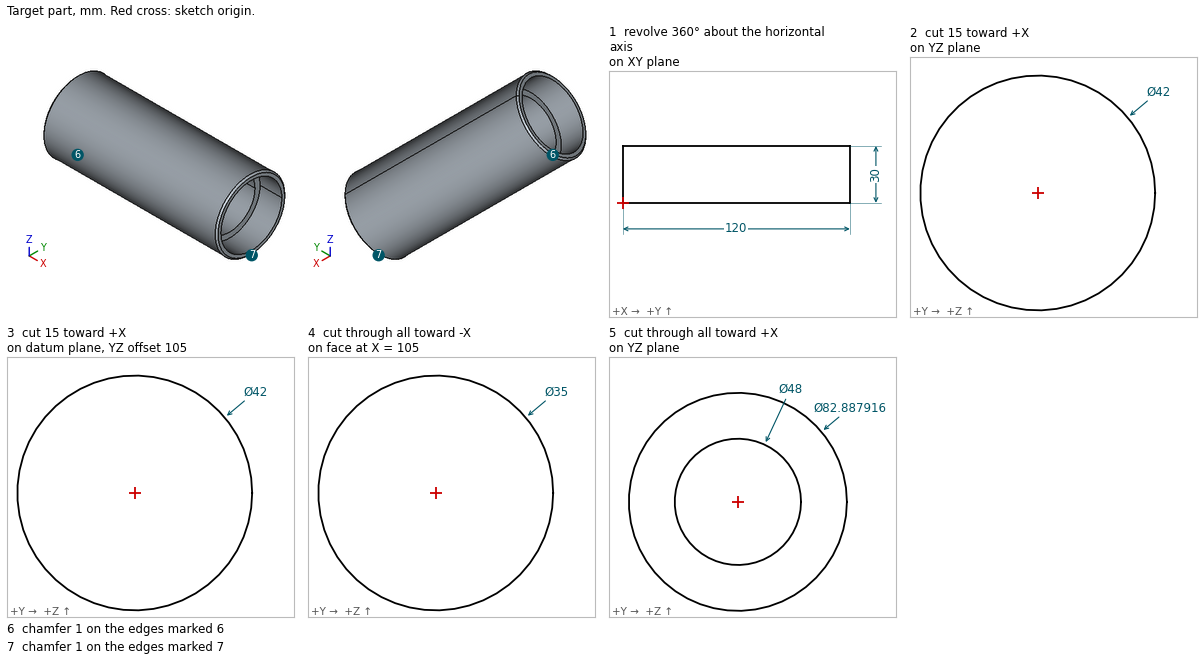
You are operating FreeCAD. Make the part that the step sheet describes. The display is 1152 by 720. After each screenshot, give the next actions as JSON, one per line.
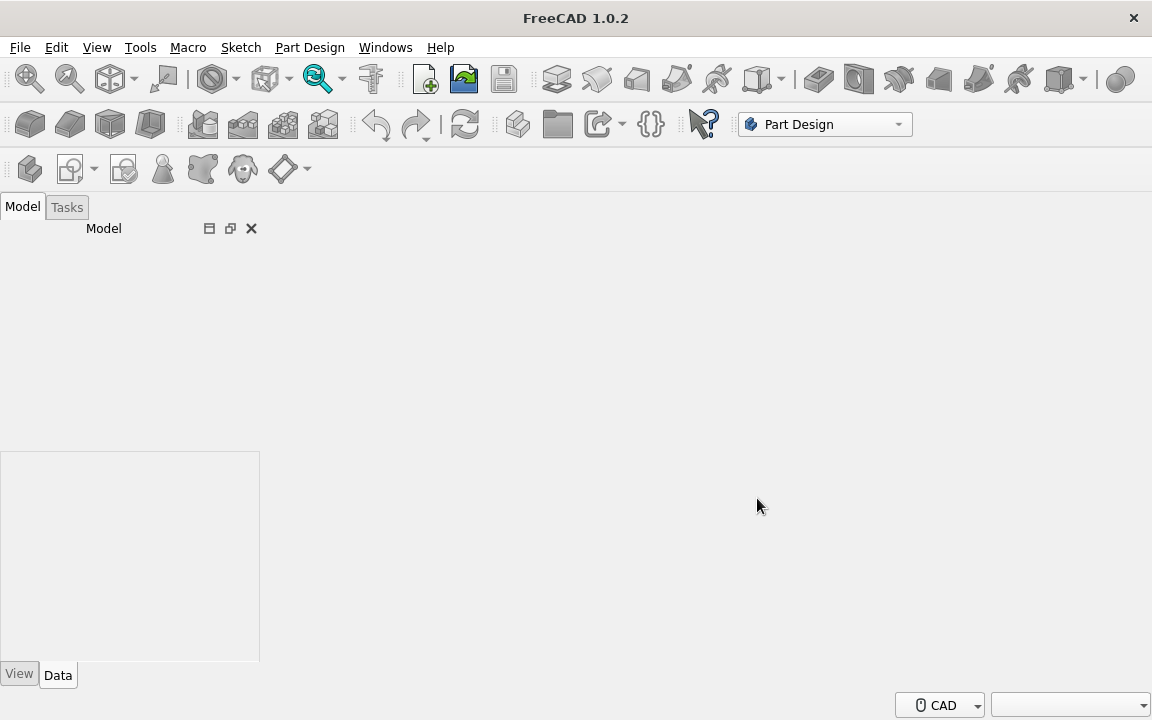
{"action": "key", "text": "ctrl+n"}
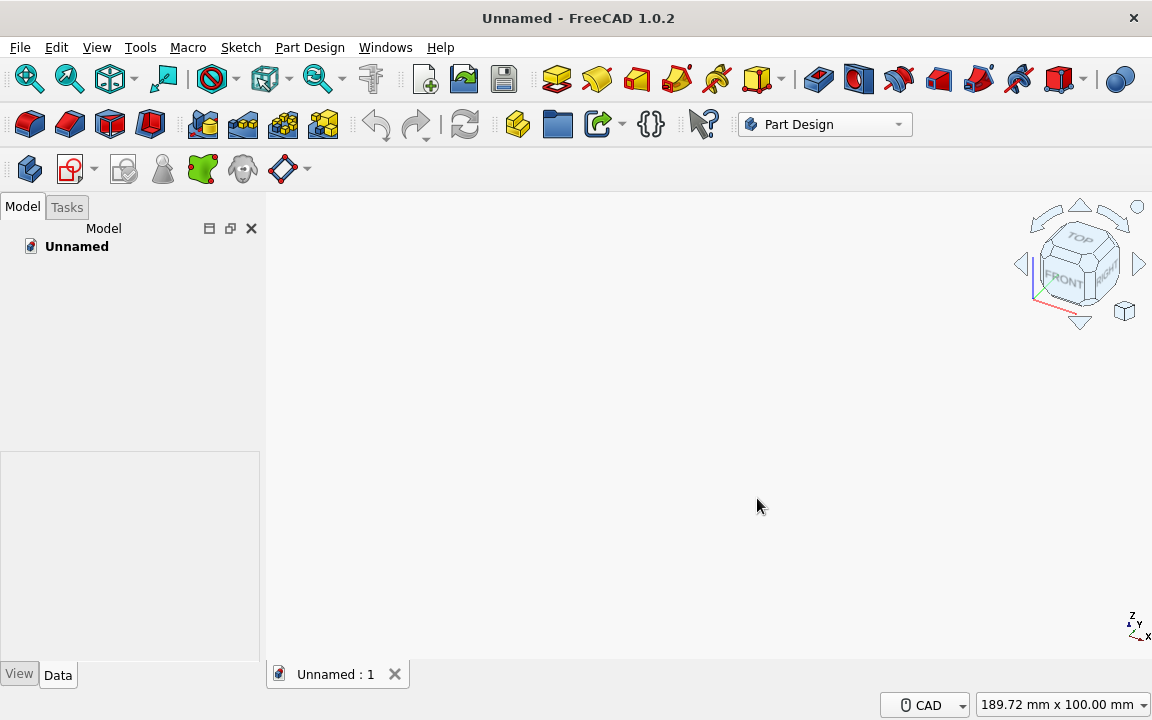
{"action": "left_click", "coordinate": [70, 170]}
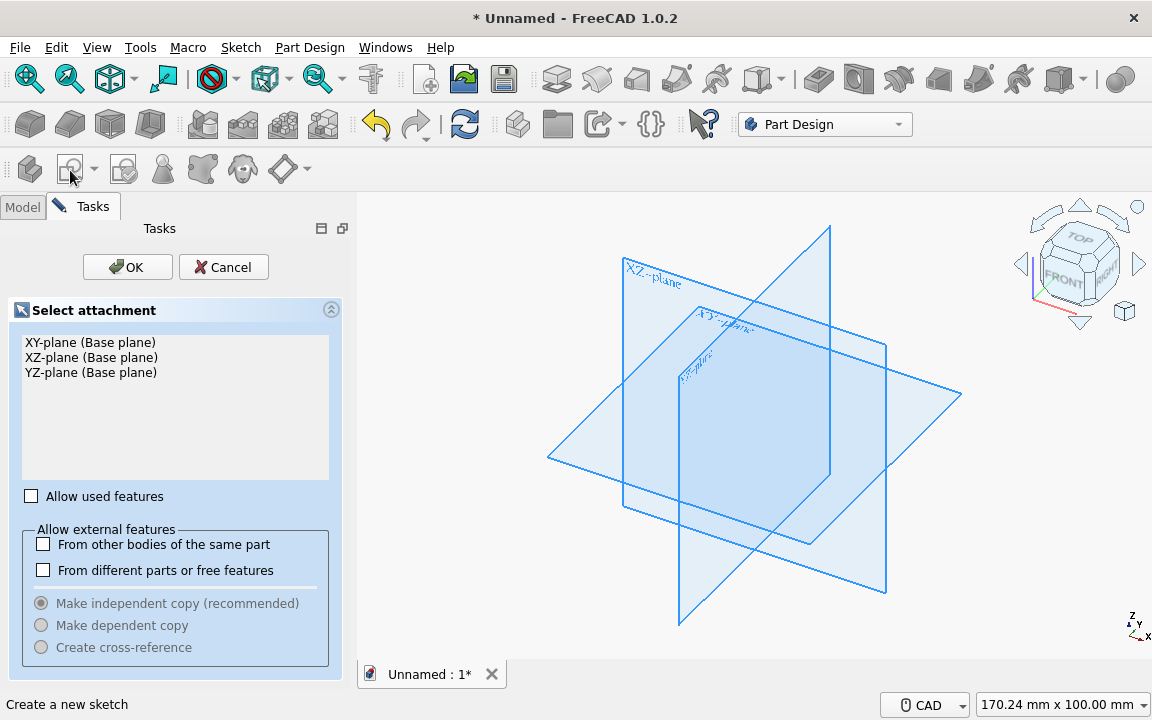
{"action": "left_click", "coordinate": [82, 342]}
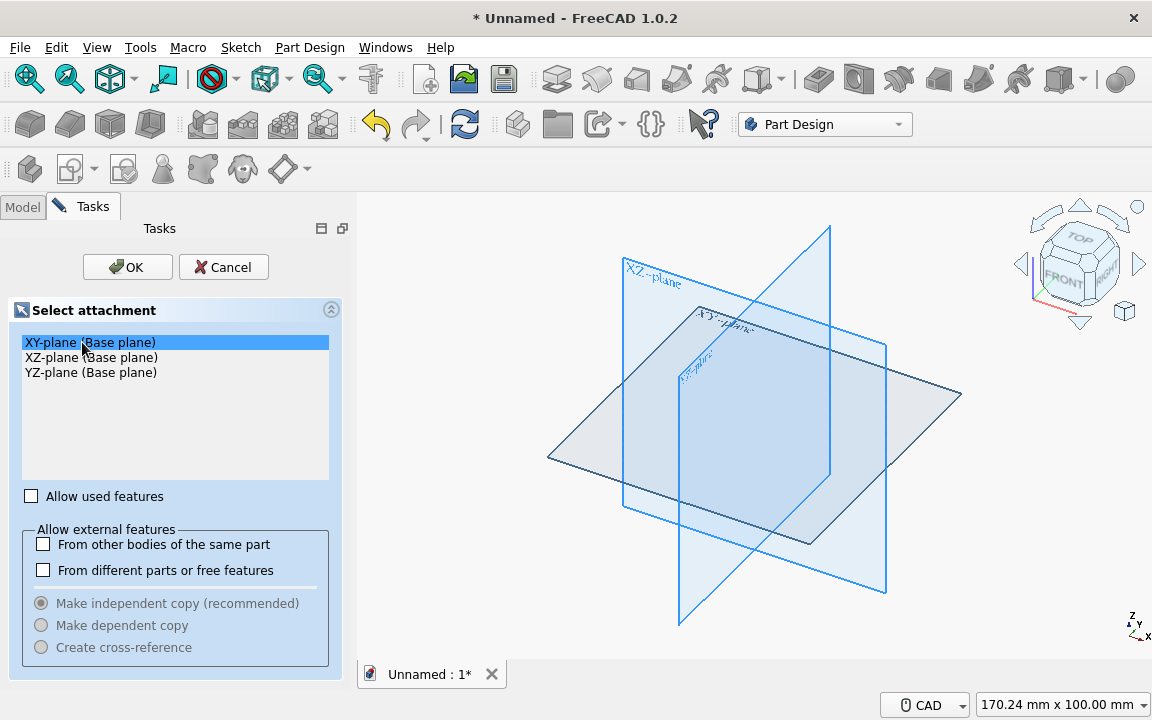
{"action": "left_click", "coordinate": [128, 267]}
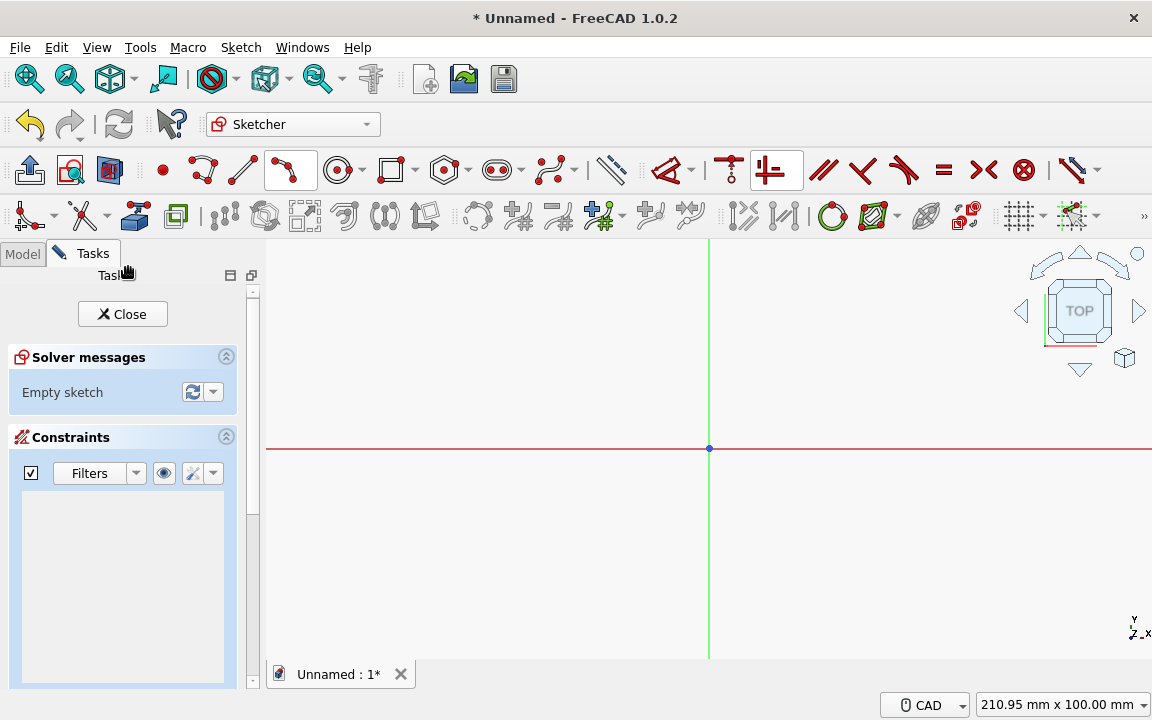
{"action": "scroll", "coordinate": [294, 577], "scroll_direction": "down", "scroll_amount": 2}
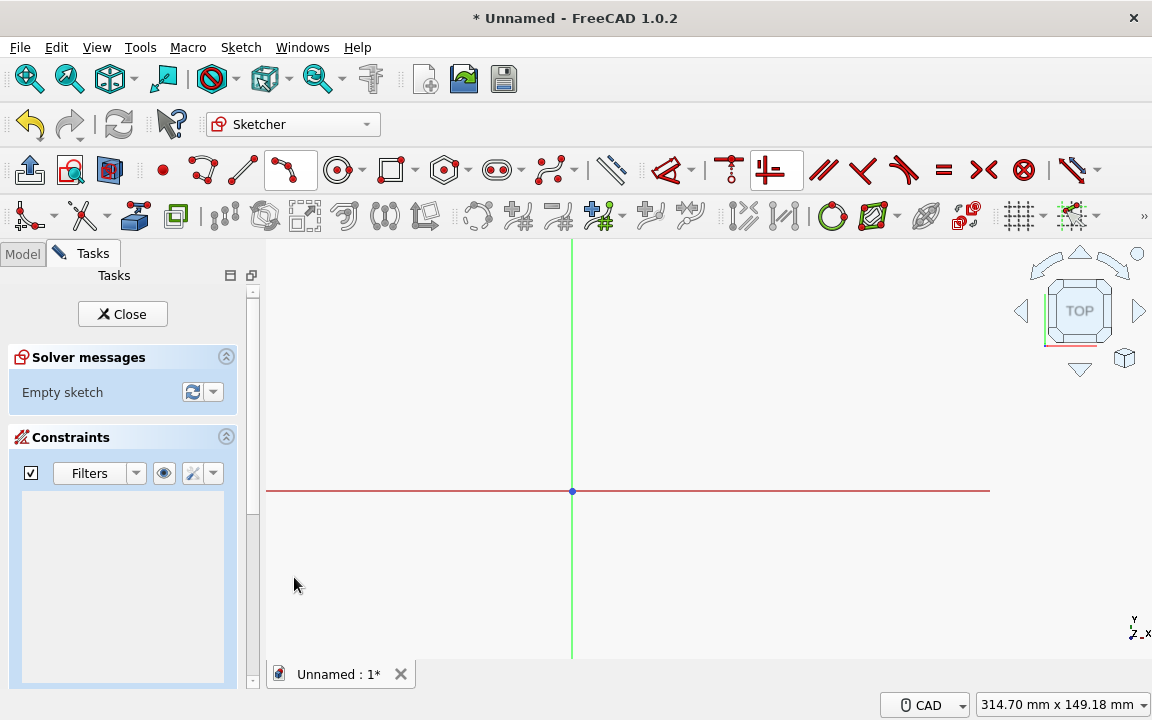
{"action": "scroll", "coordinate": [946, 450], "scroll_direction": "up", "scroll_amount": 2}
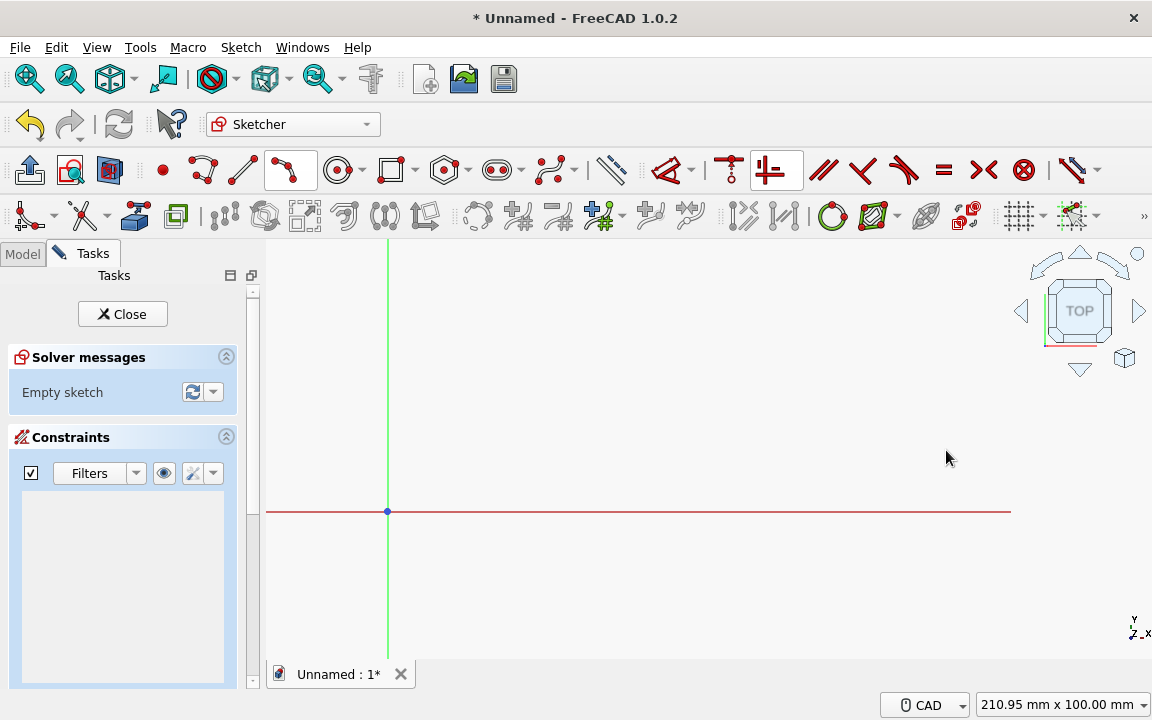
{"action": "left_click", "coordinate": [392, 170]}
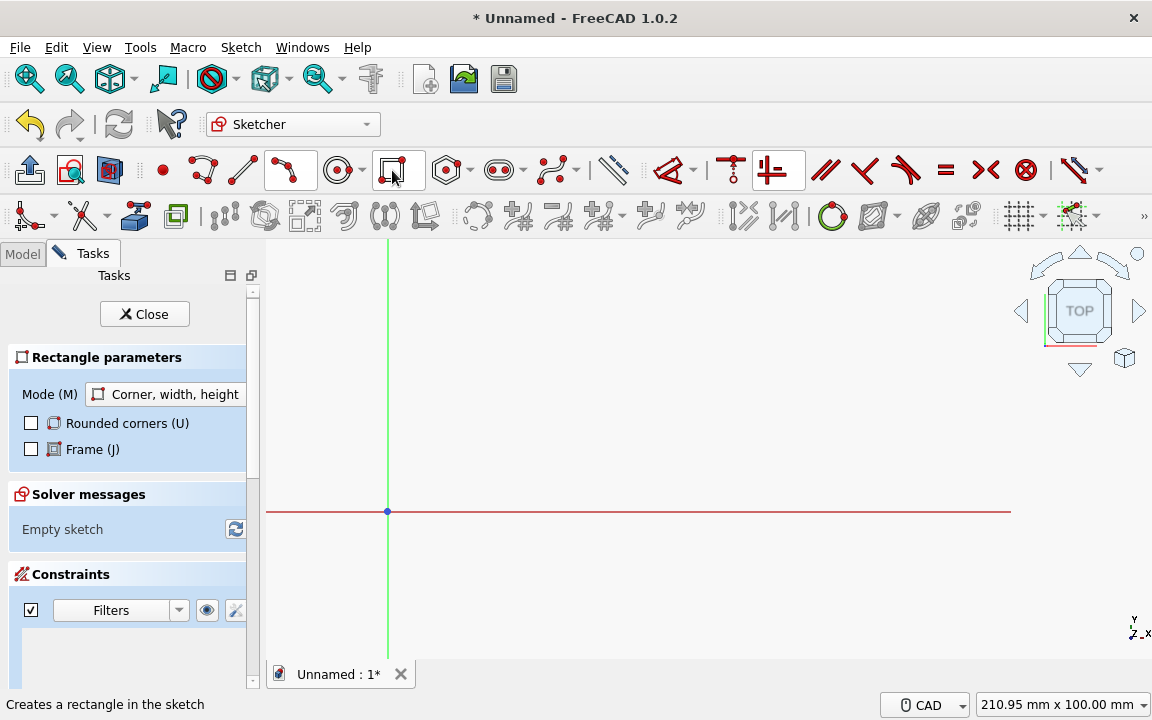
{"action": "left_click", "coordinate": [388, 512]}
{"action": "left_click", "coordinate": [892, 386]}
{"action": "key", "text": "Escape"}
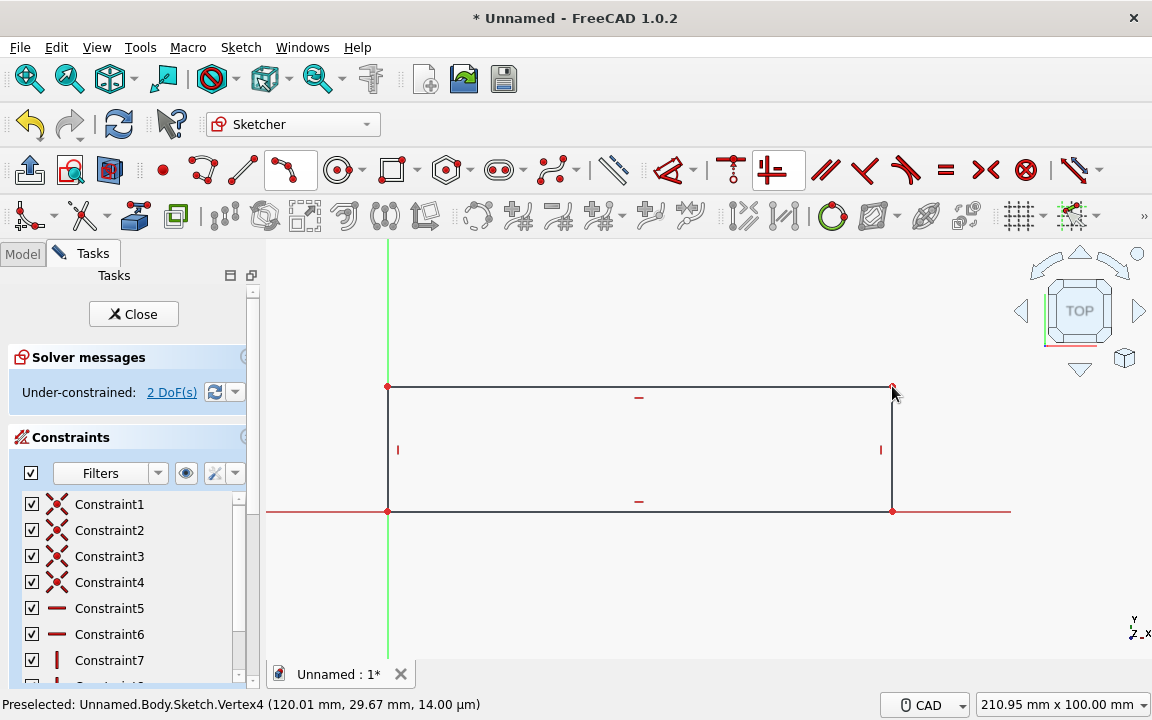
{"action": "key", "text": "d"}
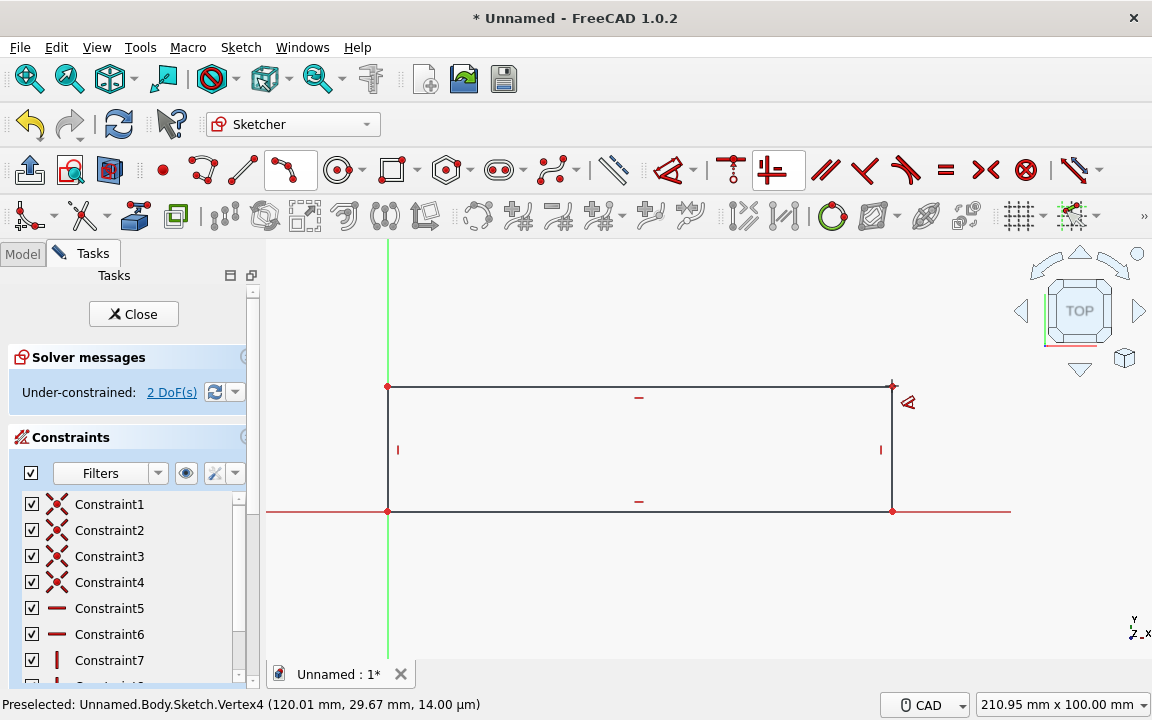
{"action": "left_click", "coordinate": [892, 474]}
{"action": "left_click", "coordinate": [926, 449]}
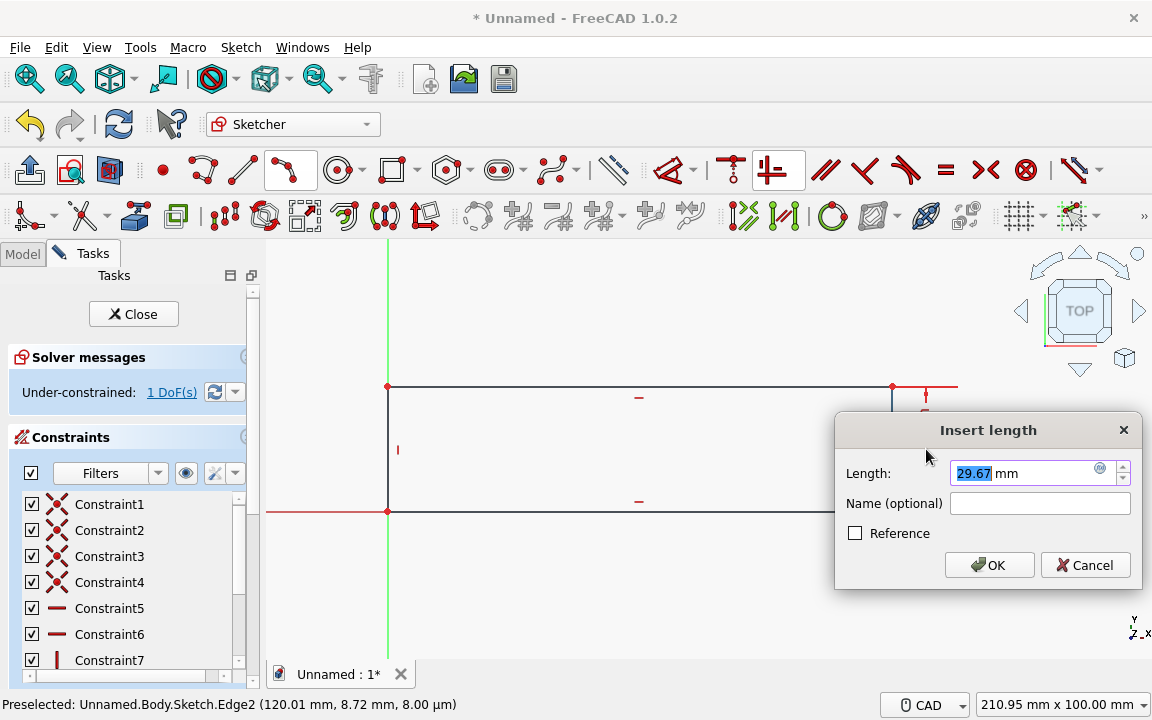
{"action": "type", "text": "30"}
{"action": "key", "text": "Return"}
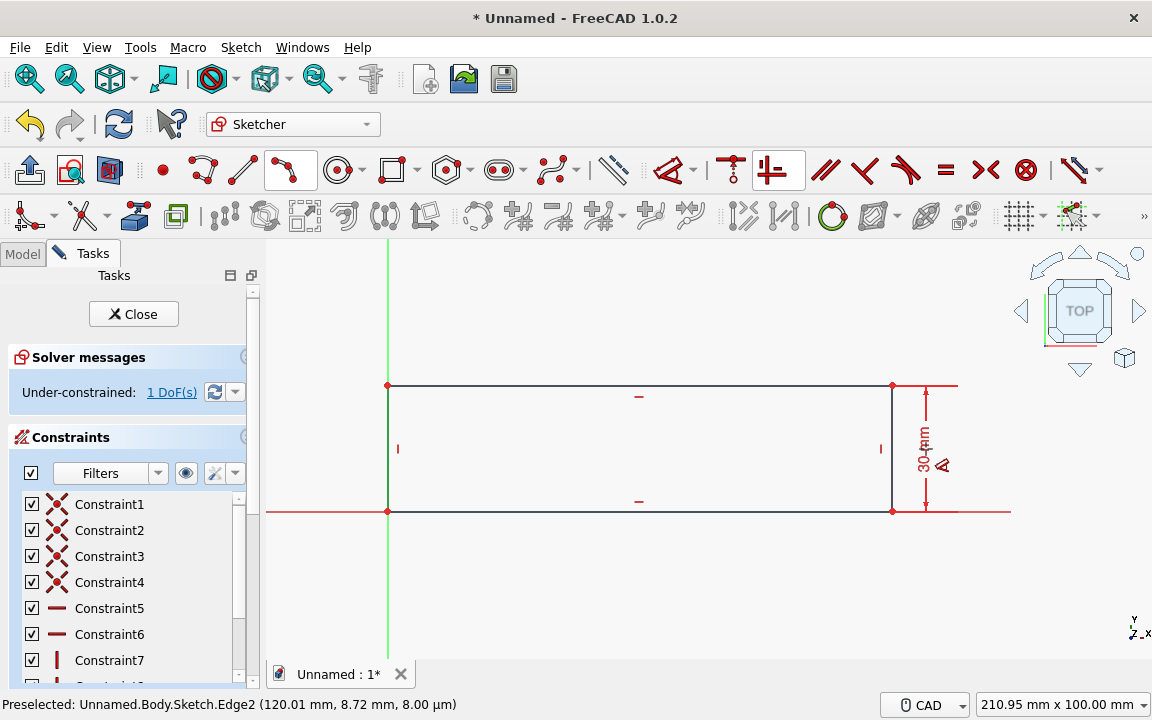
{"action": "left_click", "coordinate": [539, 512]}
{"action": "left_click", "coordinate": [640, 546]}